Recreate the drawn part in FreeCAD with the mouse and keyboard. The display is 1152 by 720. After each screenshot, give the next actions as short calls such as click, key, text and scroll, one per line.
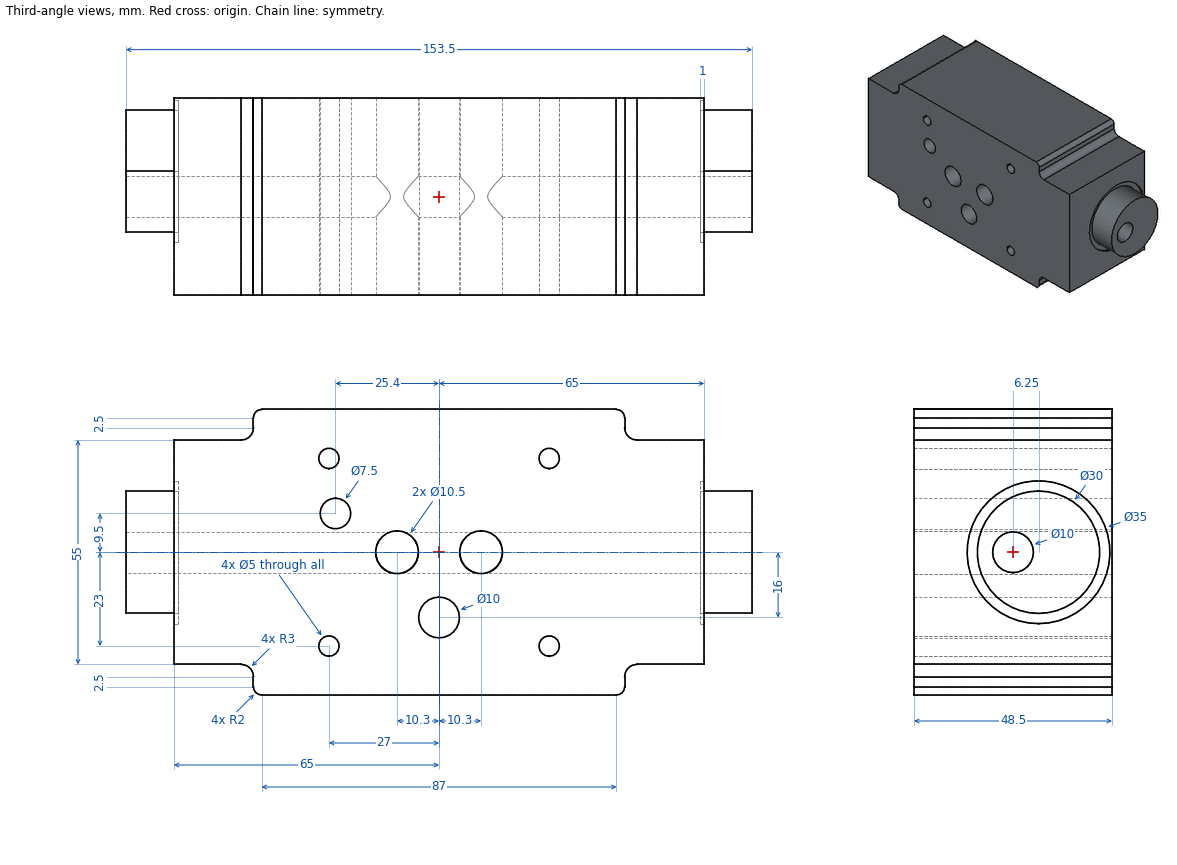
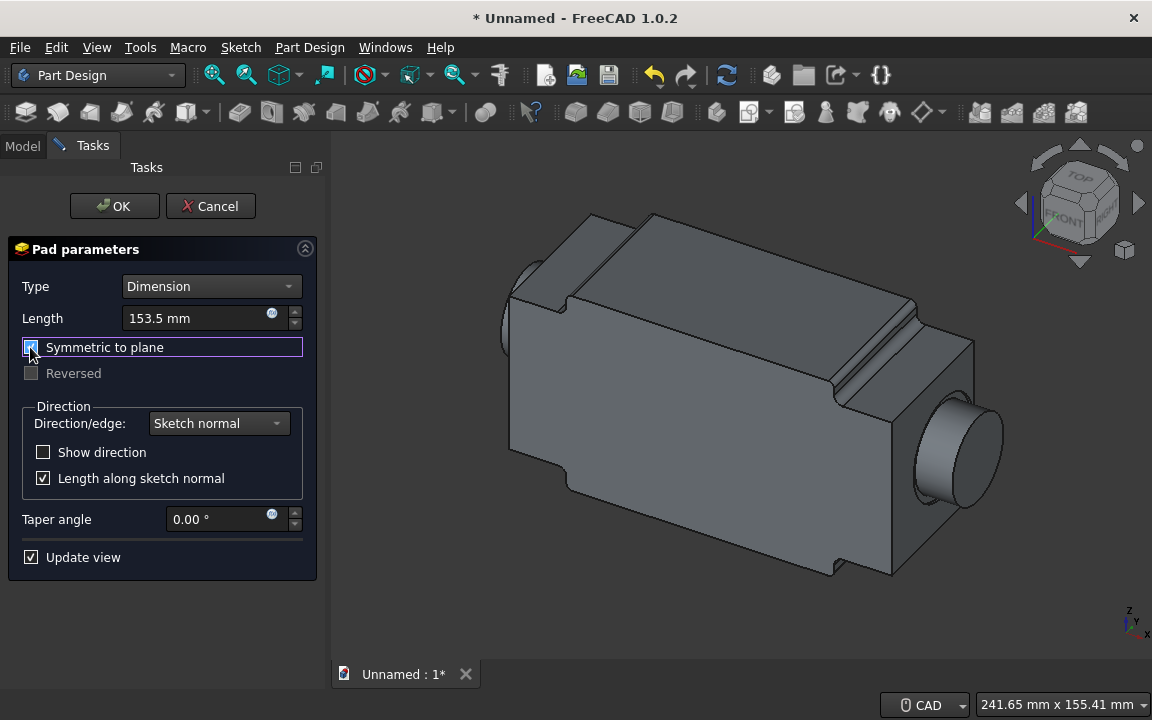
click(115, 206)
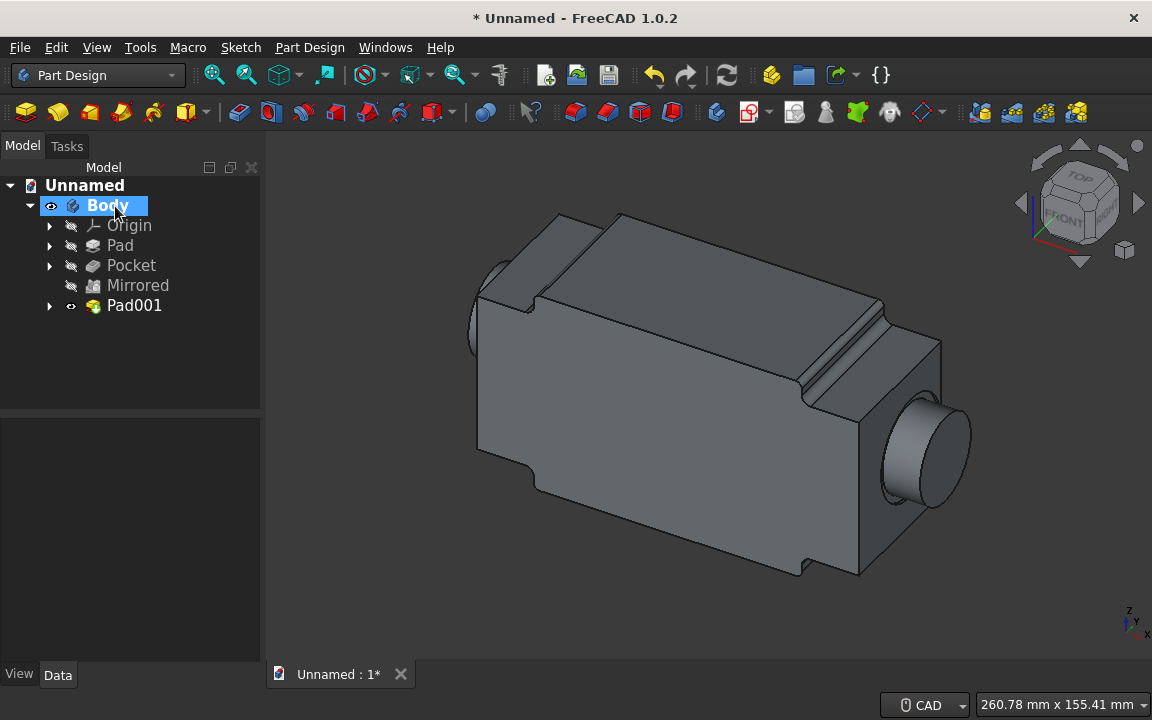
key(4)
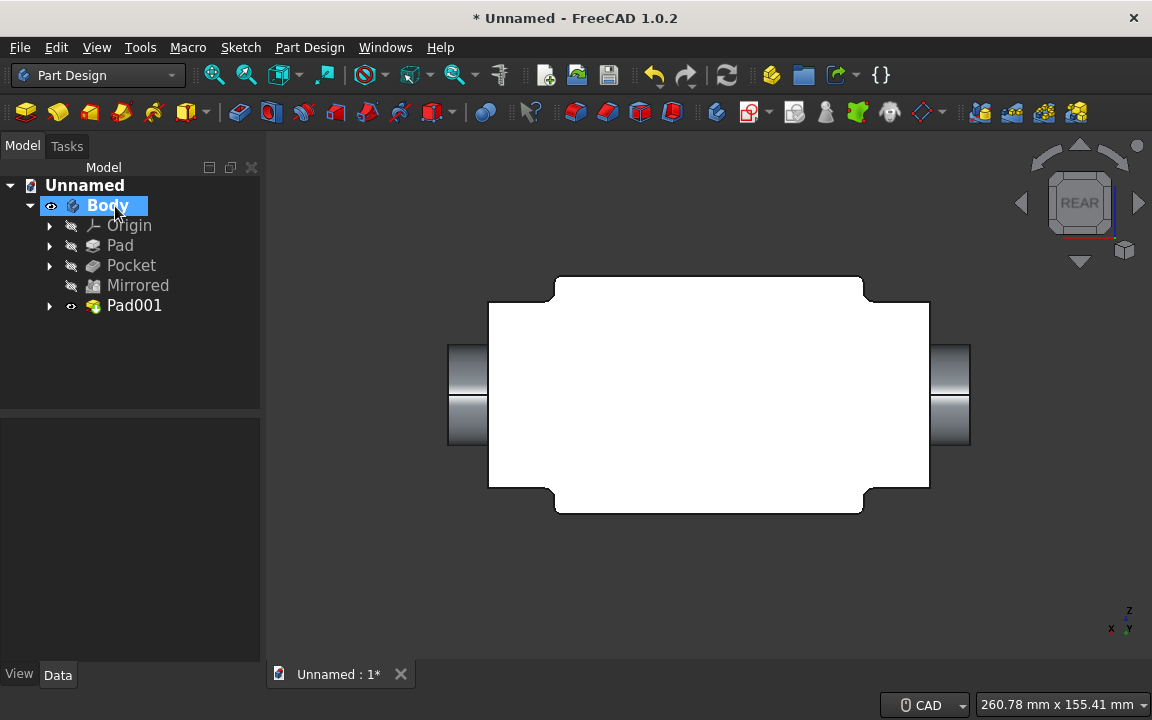
click(646, 394)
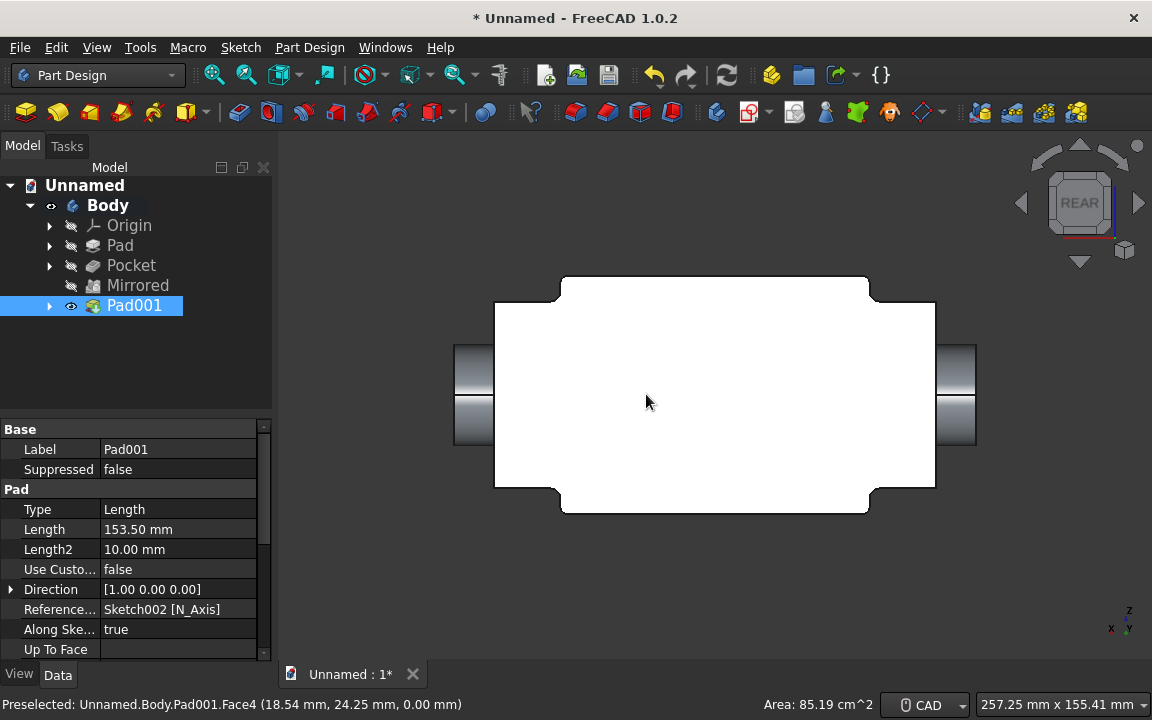
click(750, 112)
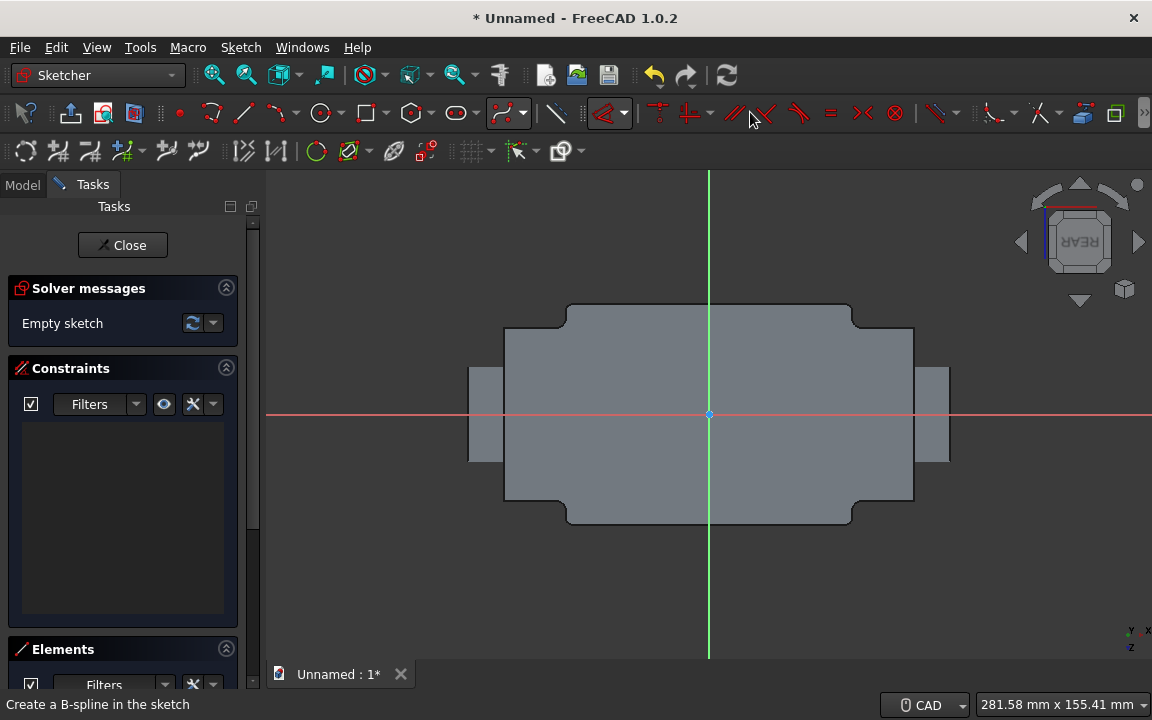
scroll(715, 395, up, 5)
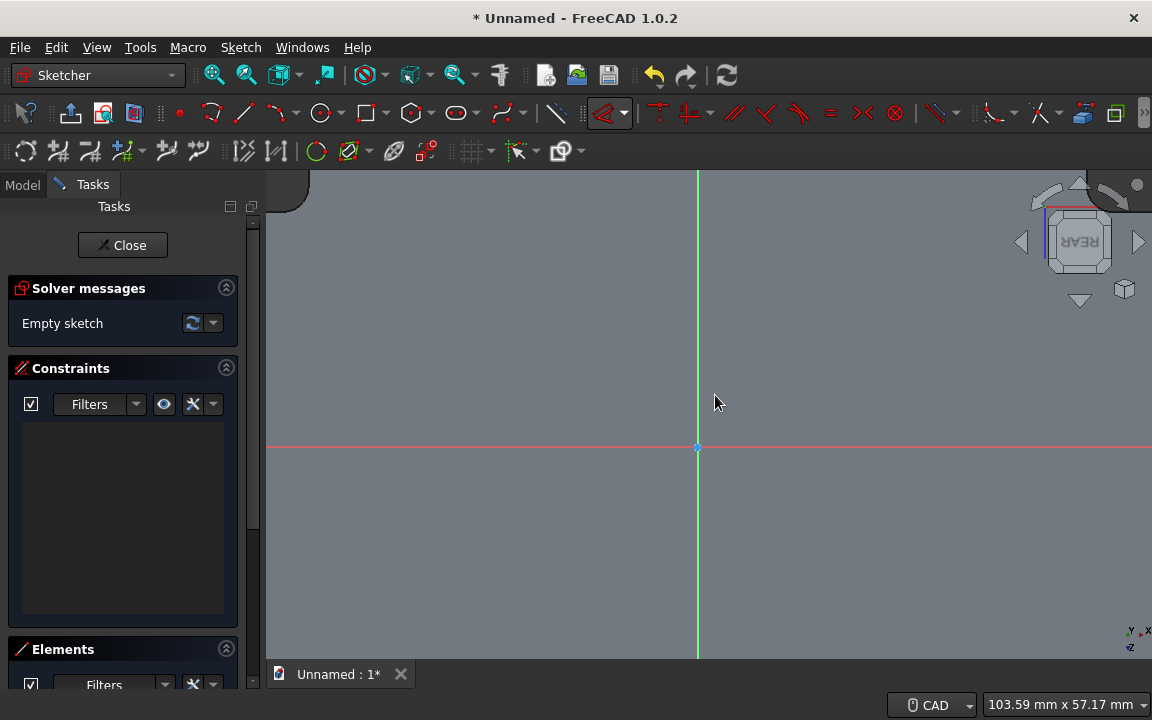
click(322, 114)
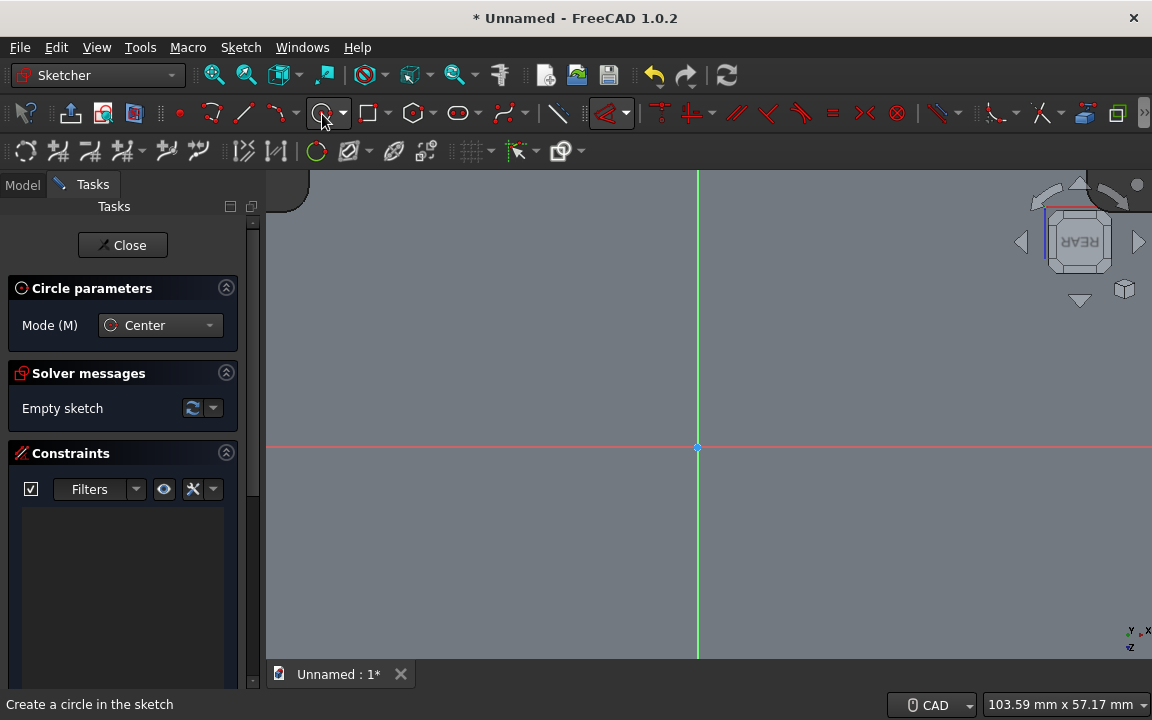
click(698, 310)
move(728, 280)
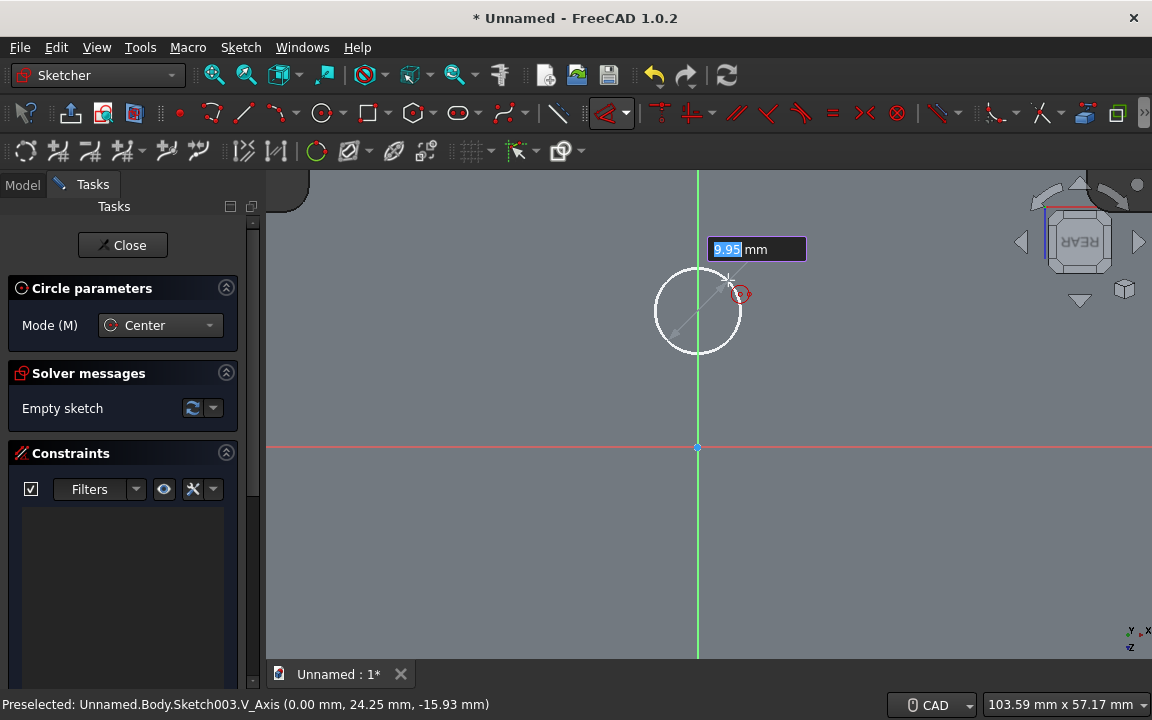
text(10)
key(Return)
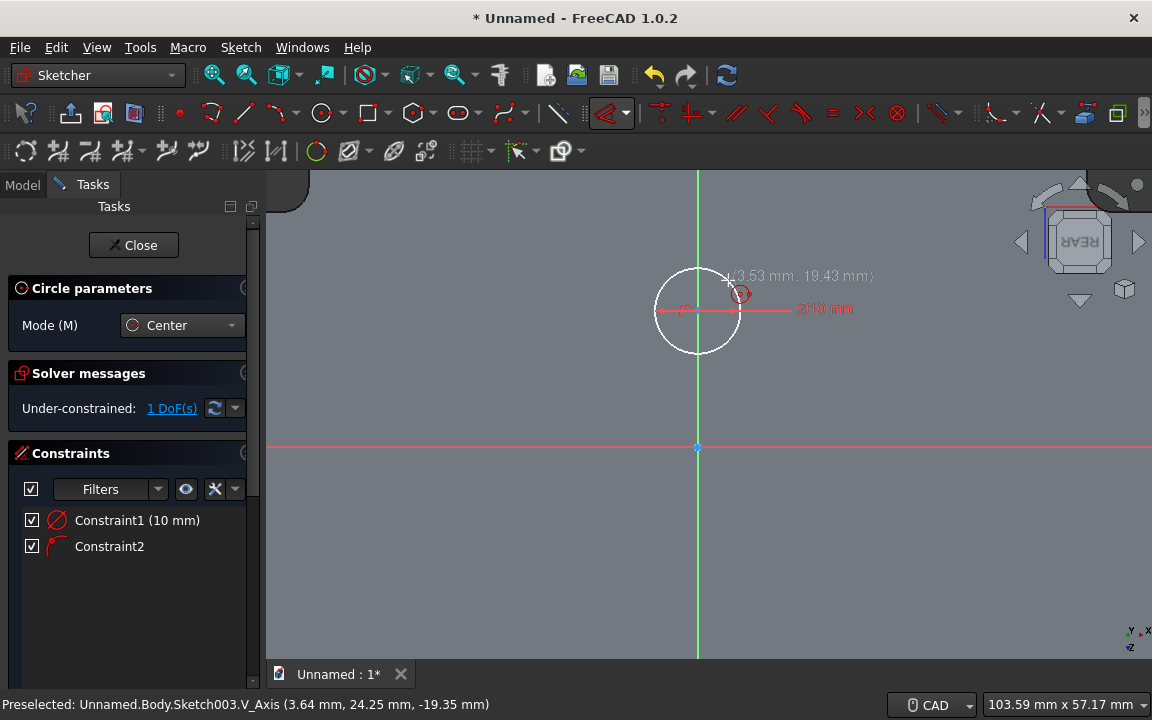
click(610, 447)
move(641, 415)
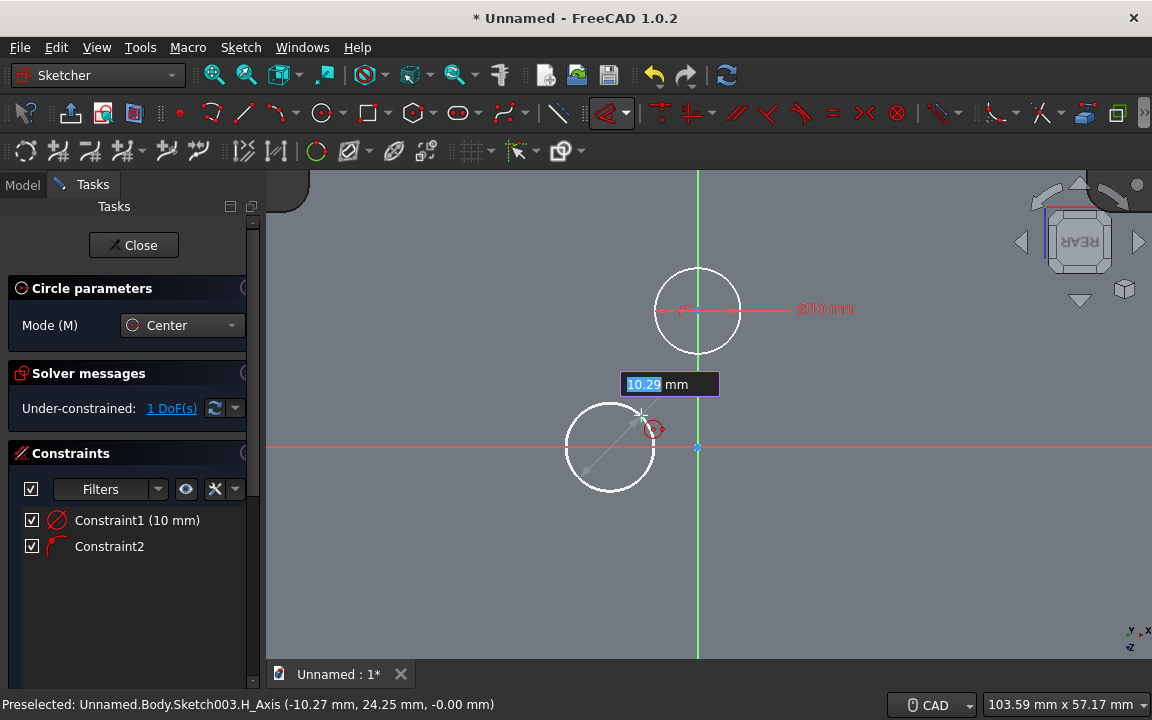
text(10.5)
key(Return)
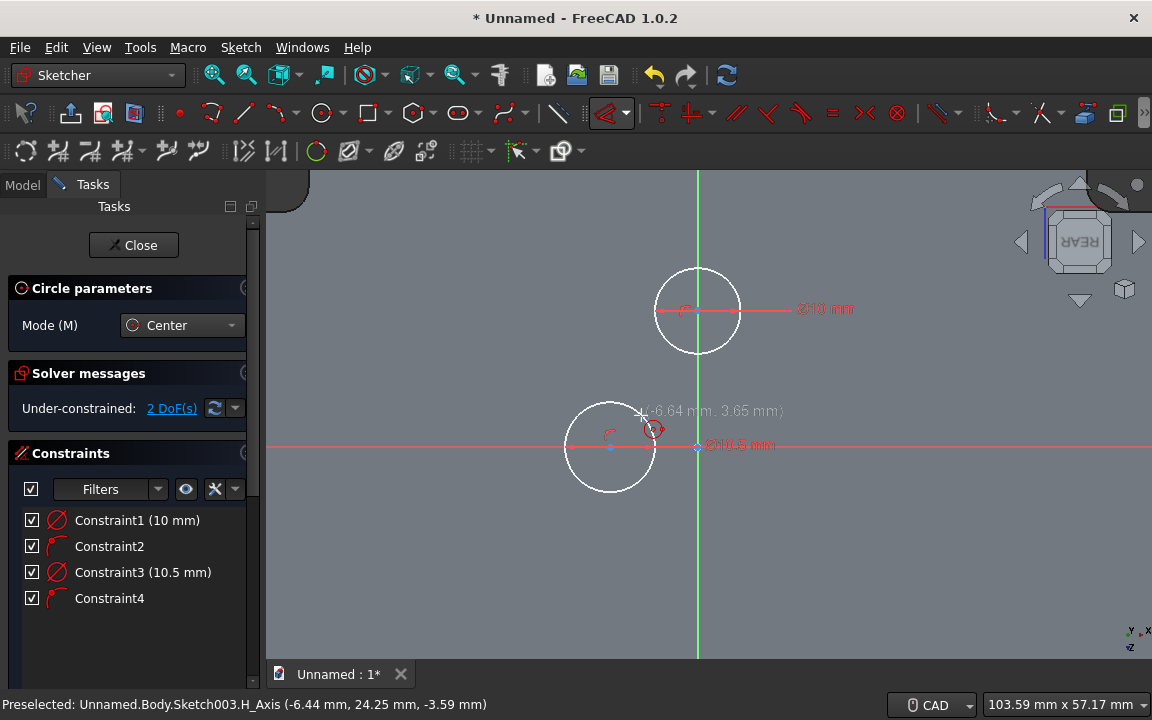
click(481, 528)
move(503, 506)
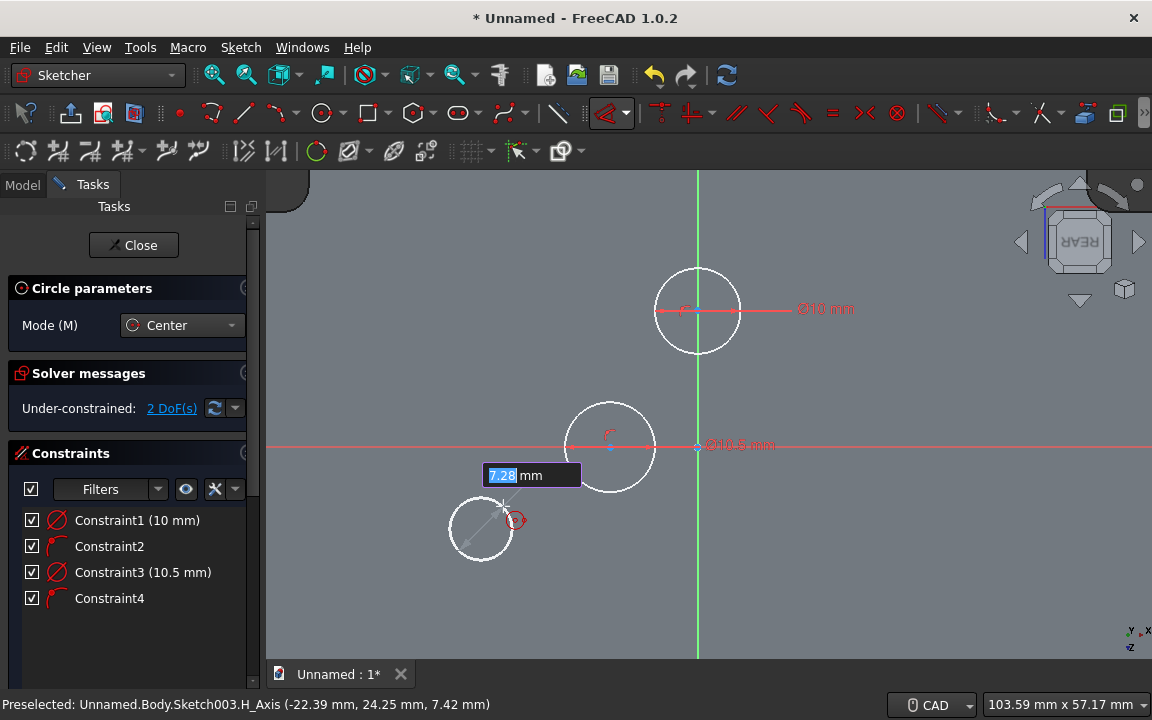
text(7.5)
key(Return)